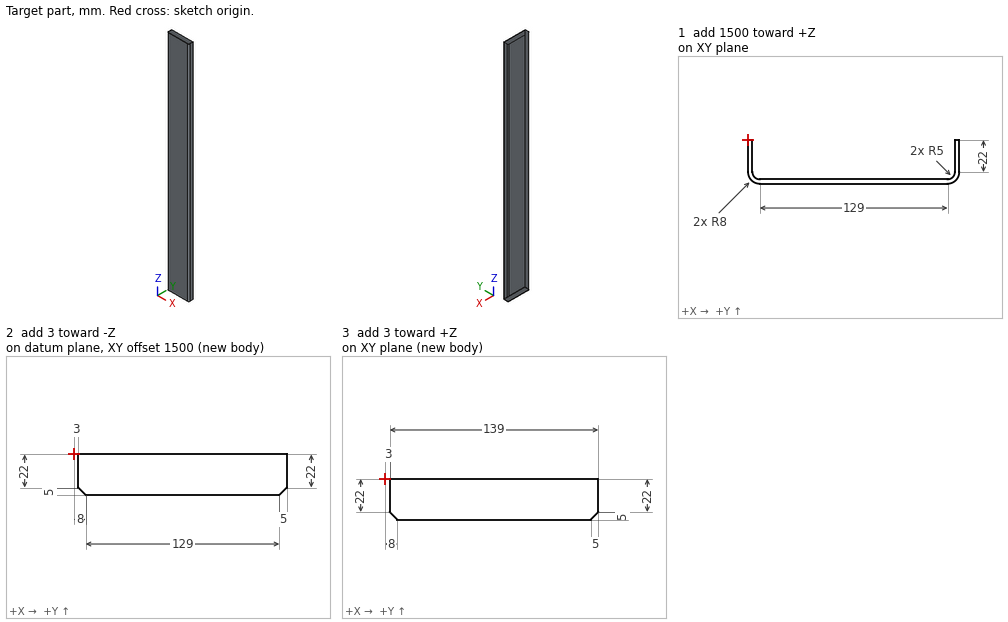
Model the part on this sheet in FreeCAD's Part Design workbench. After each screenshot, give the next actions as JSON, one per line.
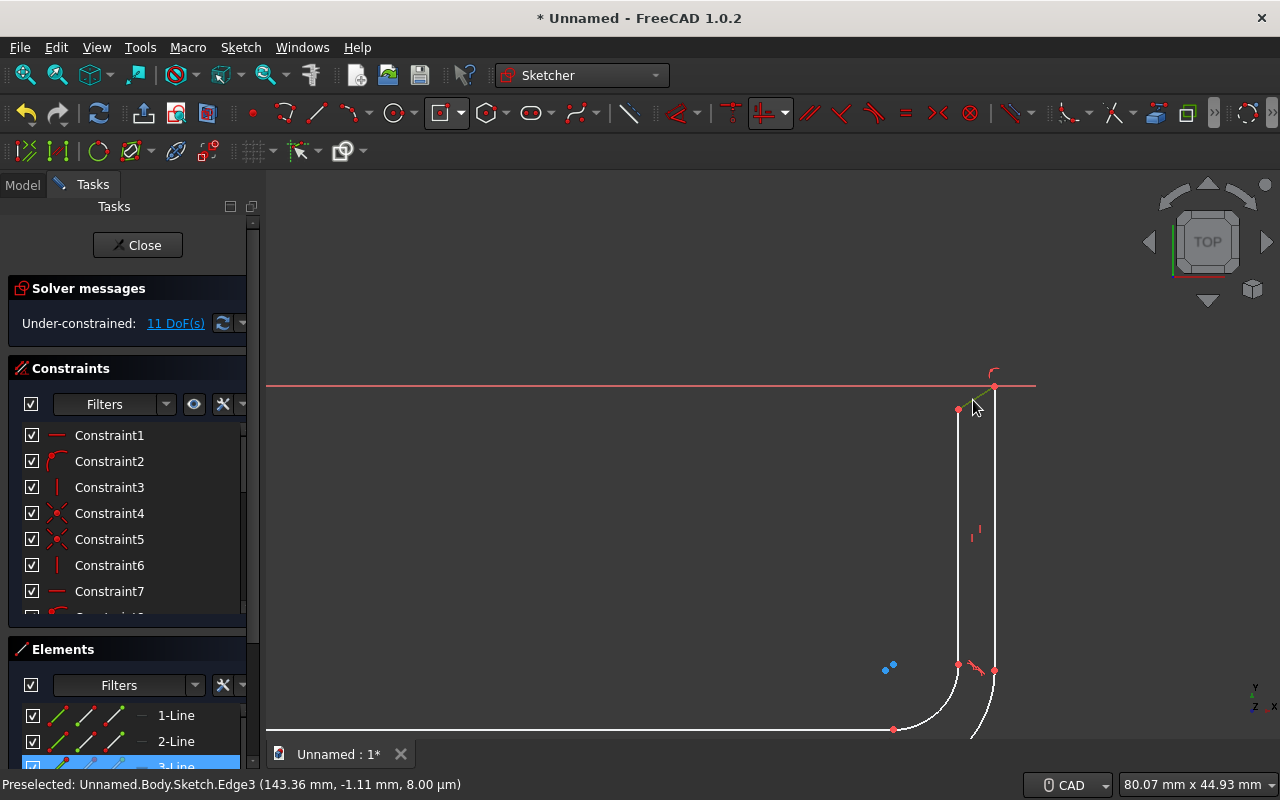
{"action": "left_click", "coordinate": [788, 114]}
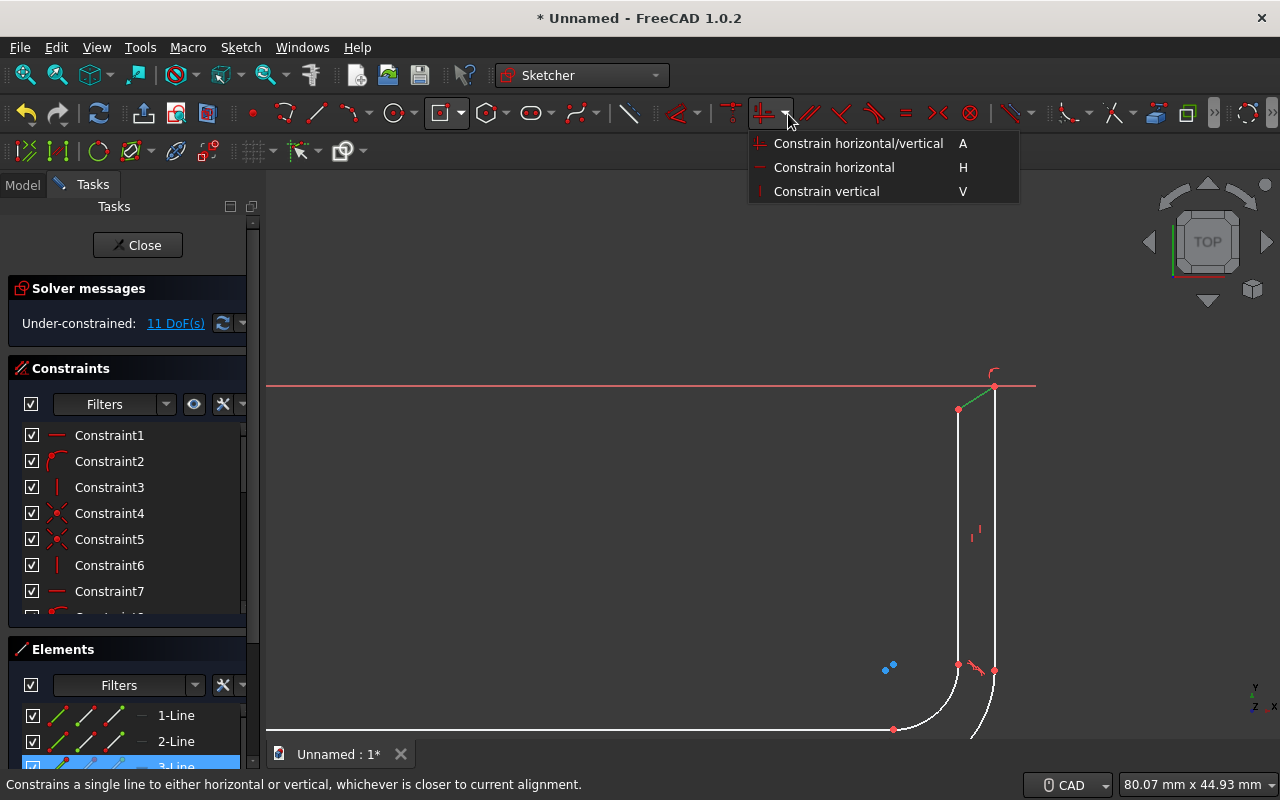
{"action": "left_click", "coordinate": [884, 167]}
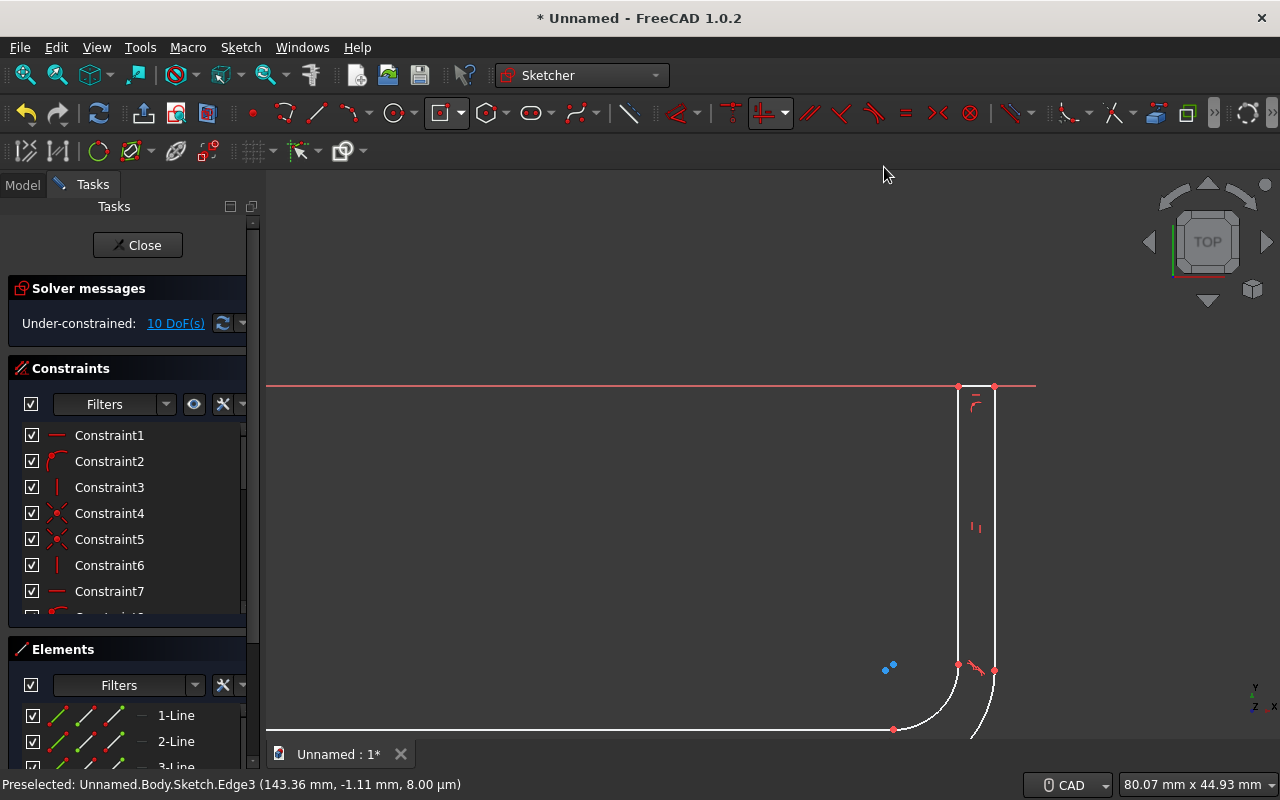
{"action": "scroll", "coordinate": [976, 402], "scroll_direction": "down", "scroll_amount": 6}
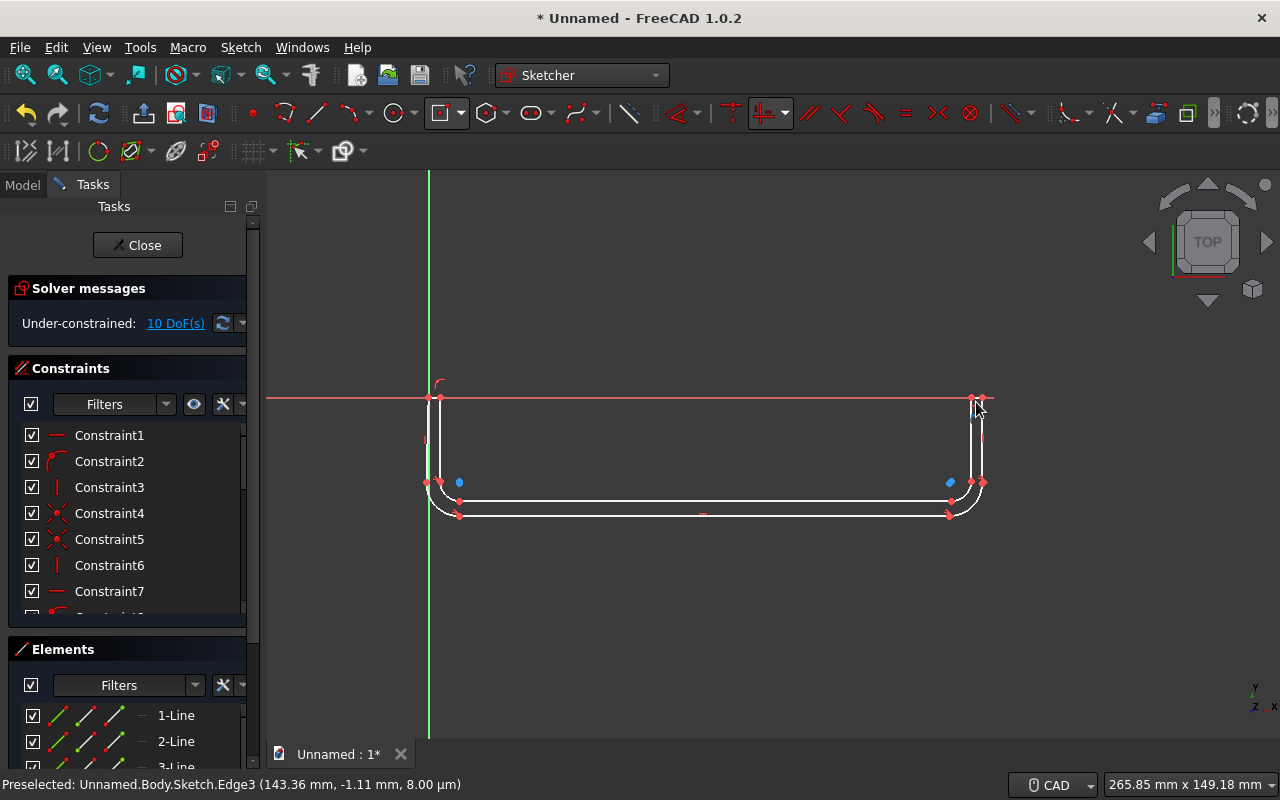
{"action": "left_click", "coordinate": [428, 423]}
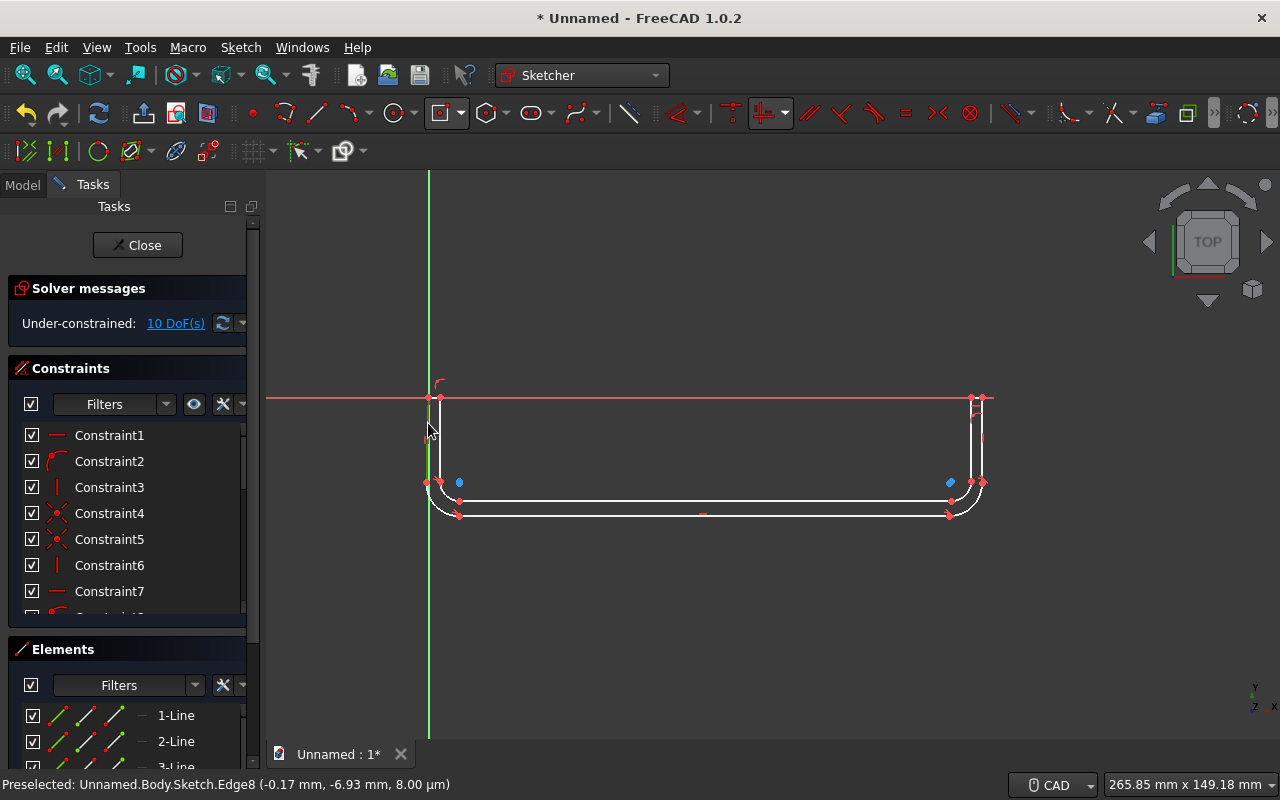
{"action": "key", "text": "v"}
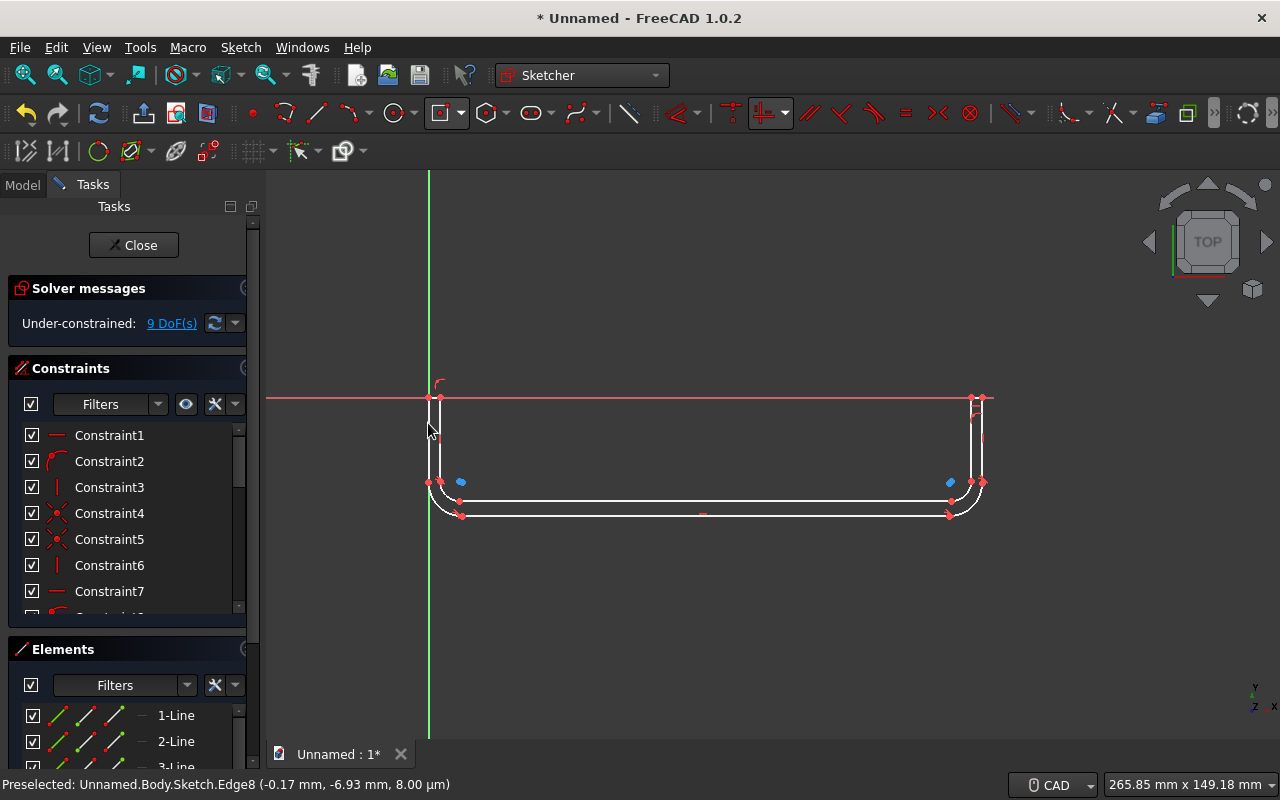
{"action": "left_click", "coordinate": [964, 513]}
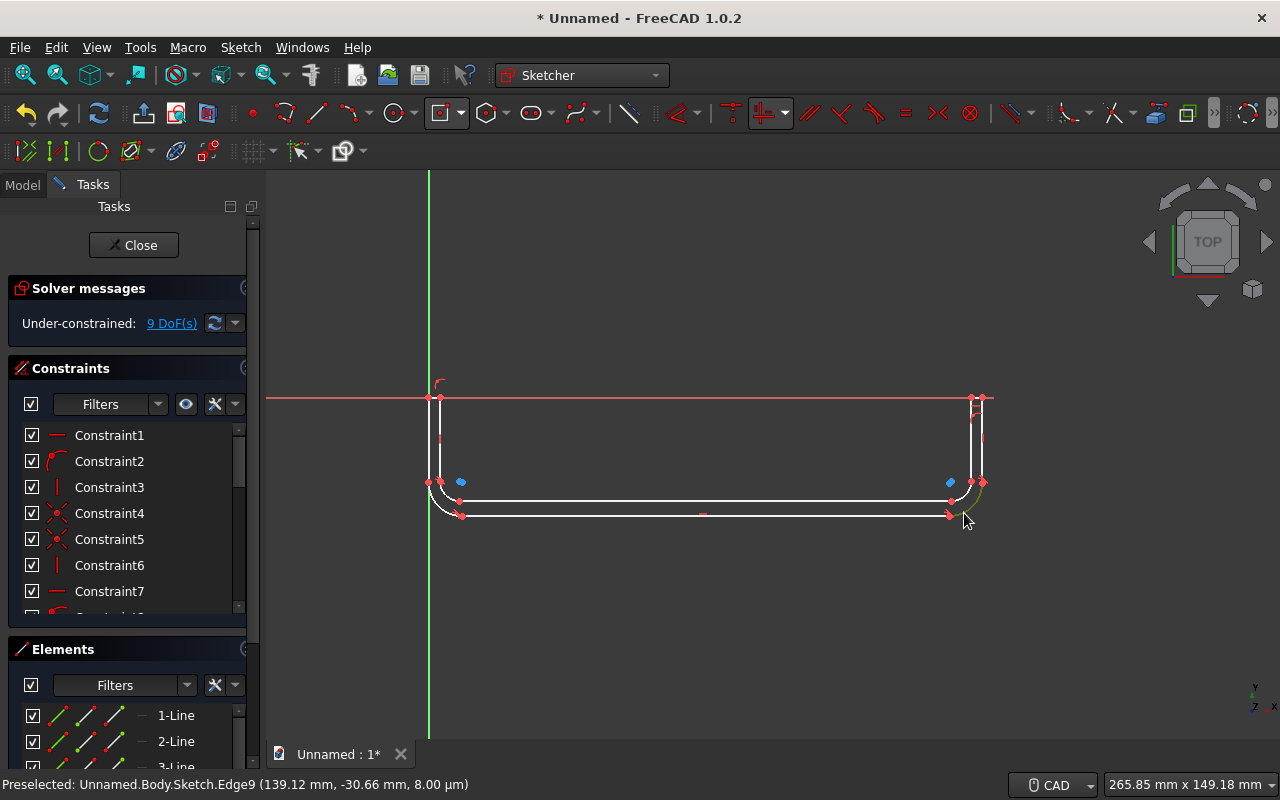
{"action": "scroll", "coordinate": [960, 499], "scroll_direction": "up", "scroll_amount": 3}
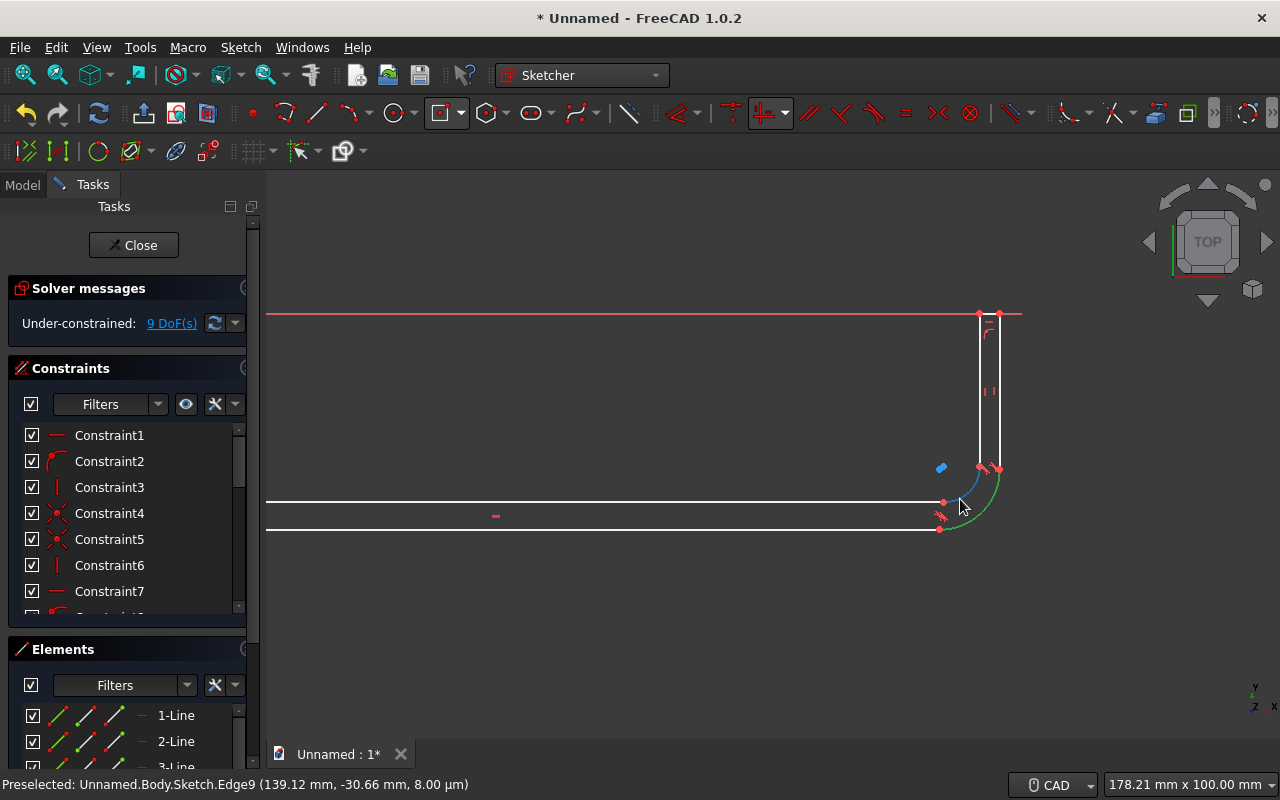
{"action": "left_click", "coordinate": [960, 498]}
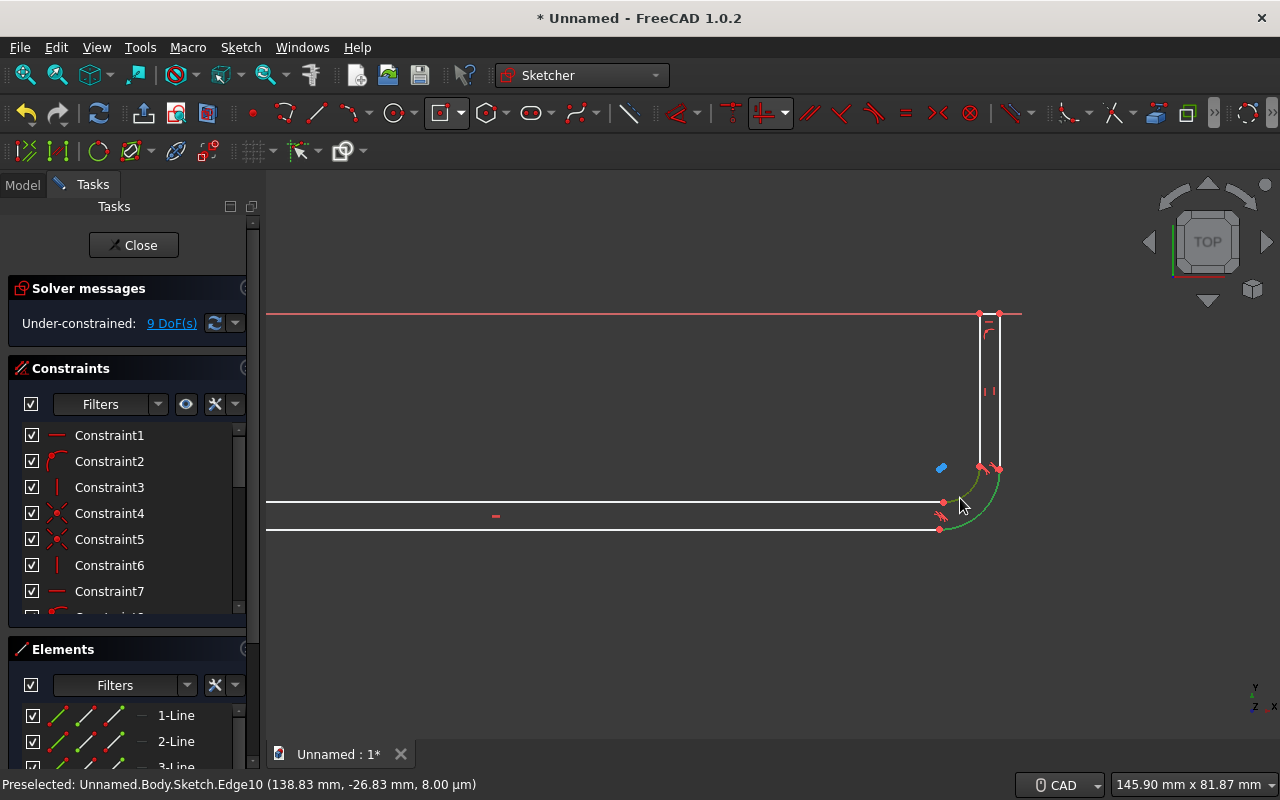
{"action": "key", "text": "c"}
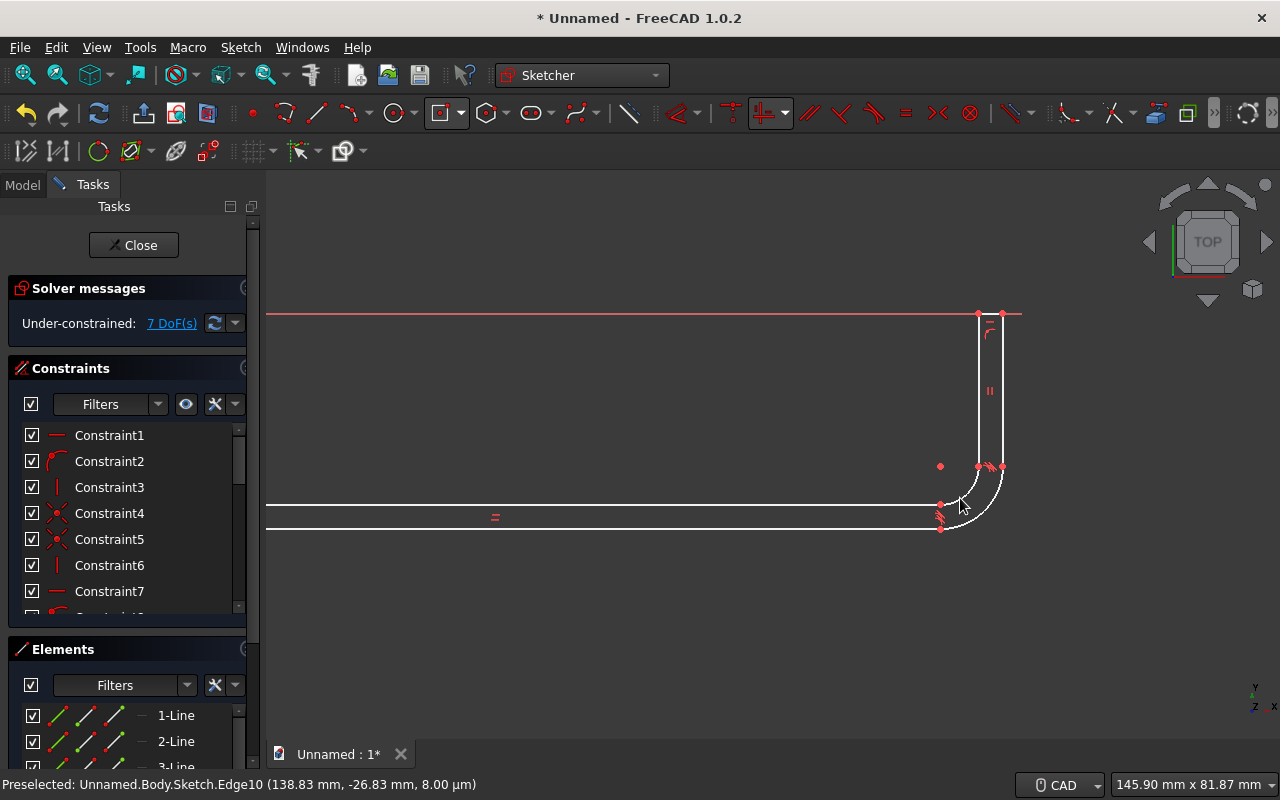
{"action": "scroll", "coordinate": [959, 499], "scroll_direction": "down", "scroll_amount": 3}